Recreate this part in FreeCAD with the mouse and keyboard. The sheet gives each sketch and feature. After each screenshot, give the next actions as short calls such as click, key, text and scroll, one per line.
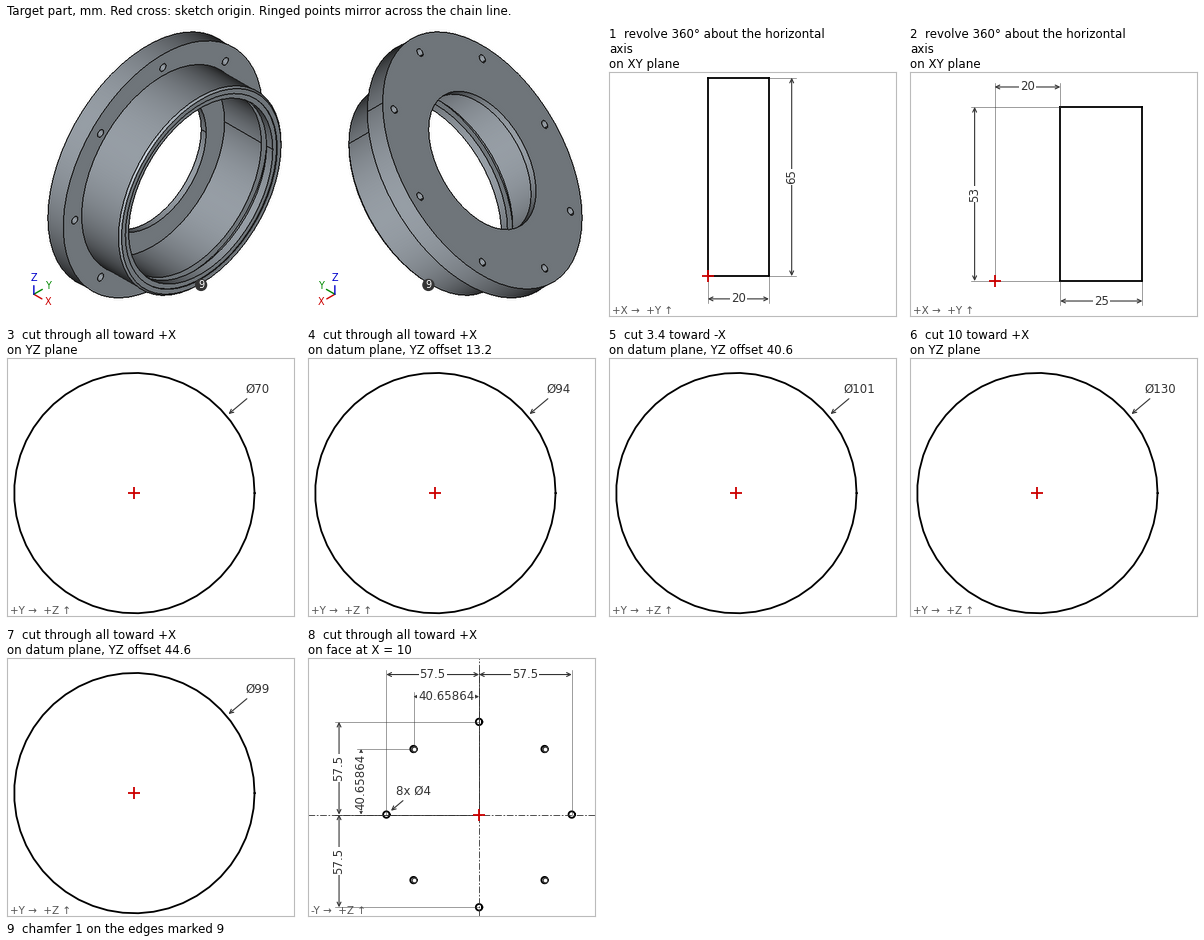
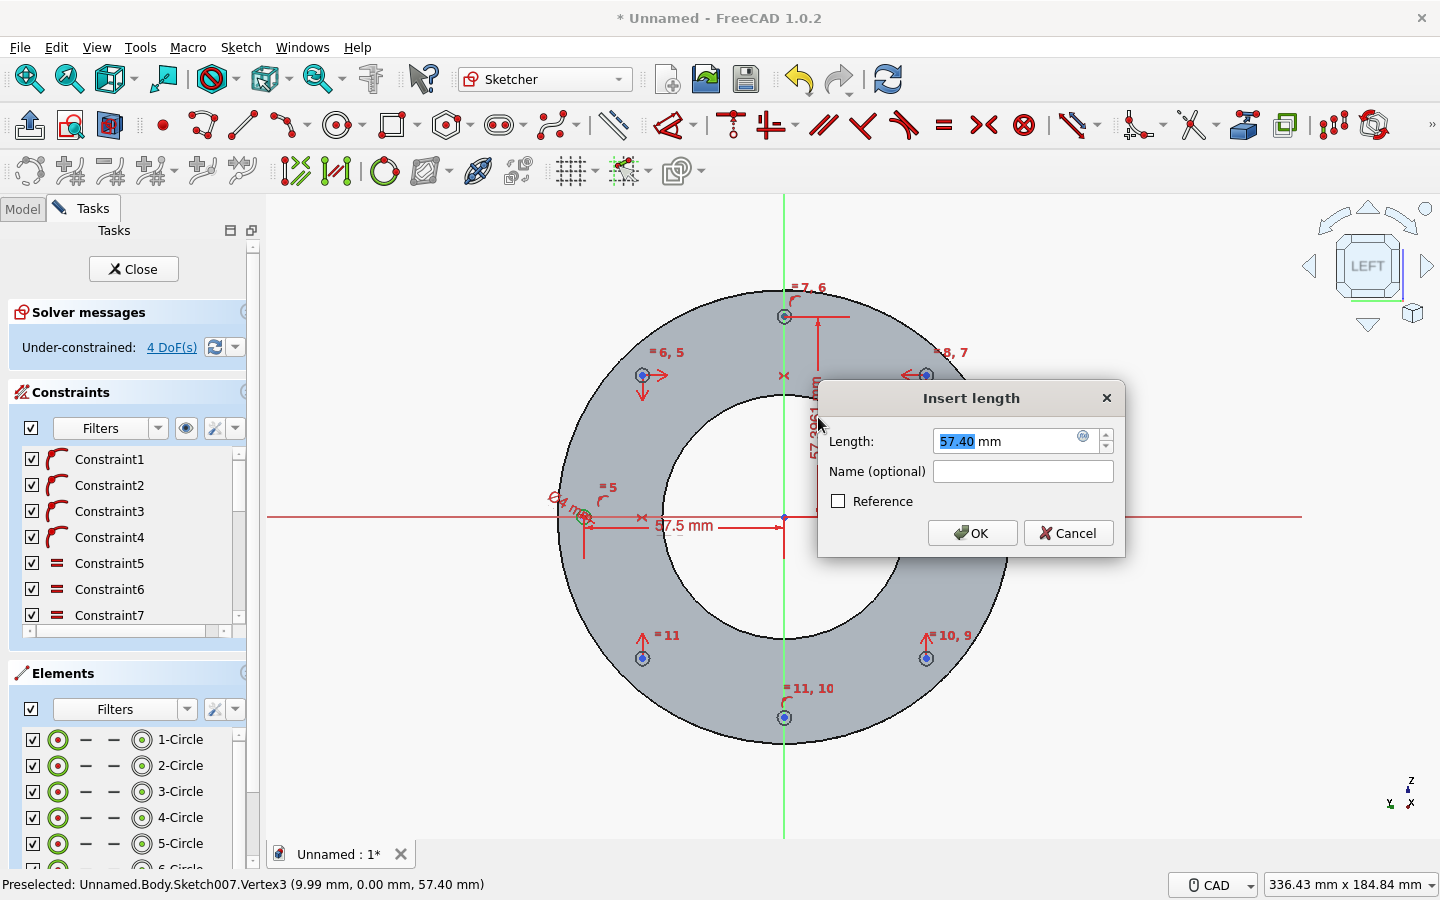
text(57.5)
key(Return)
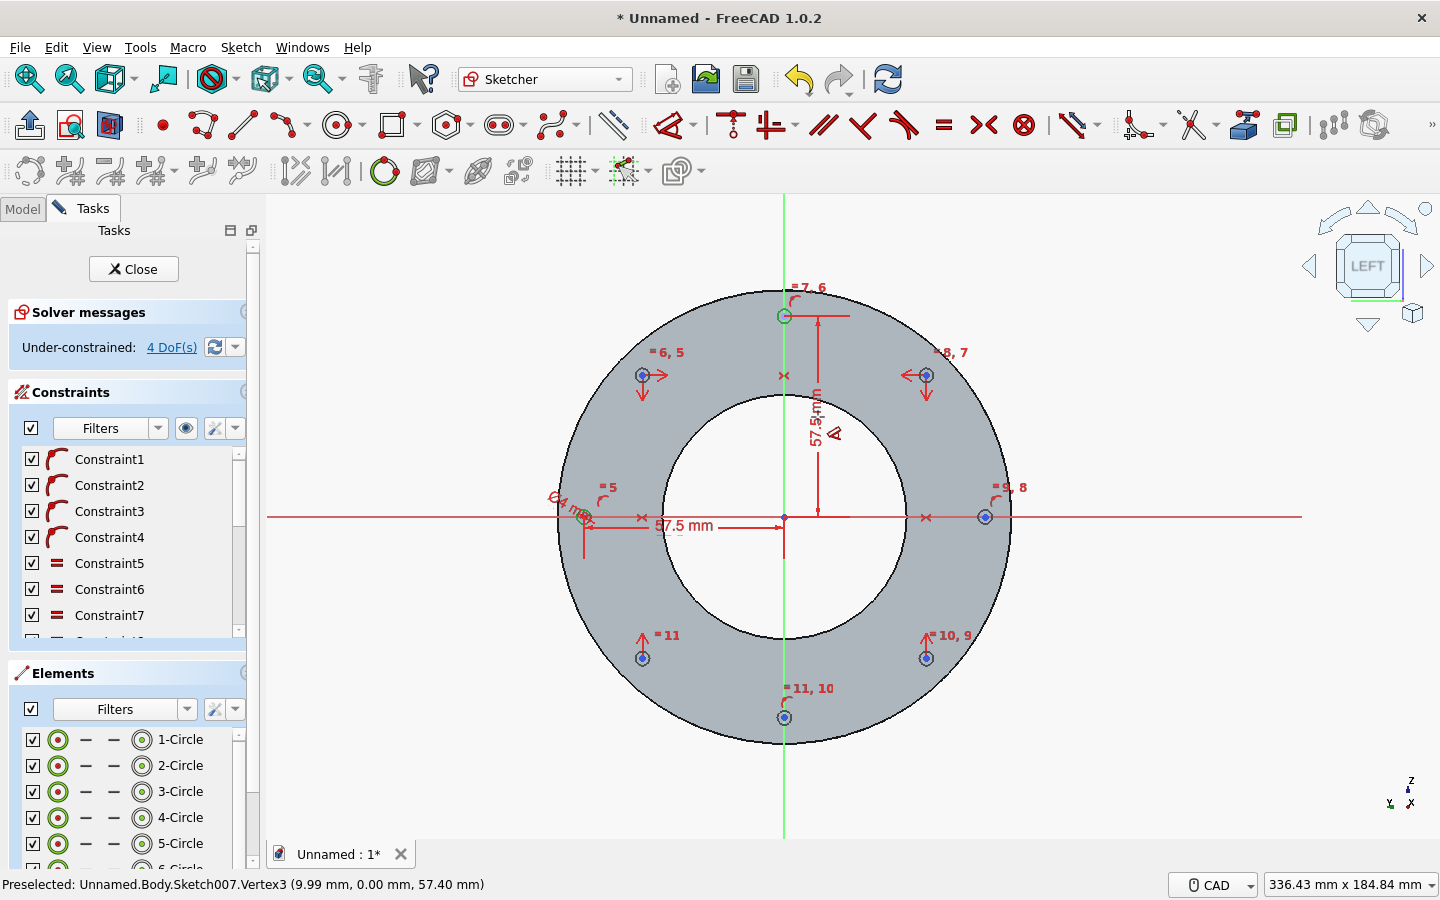
click(985, 517)
click(885, 551)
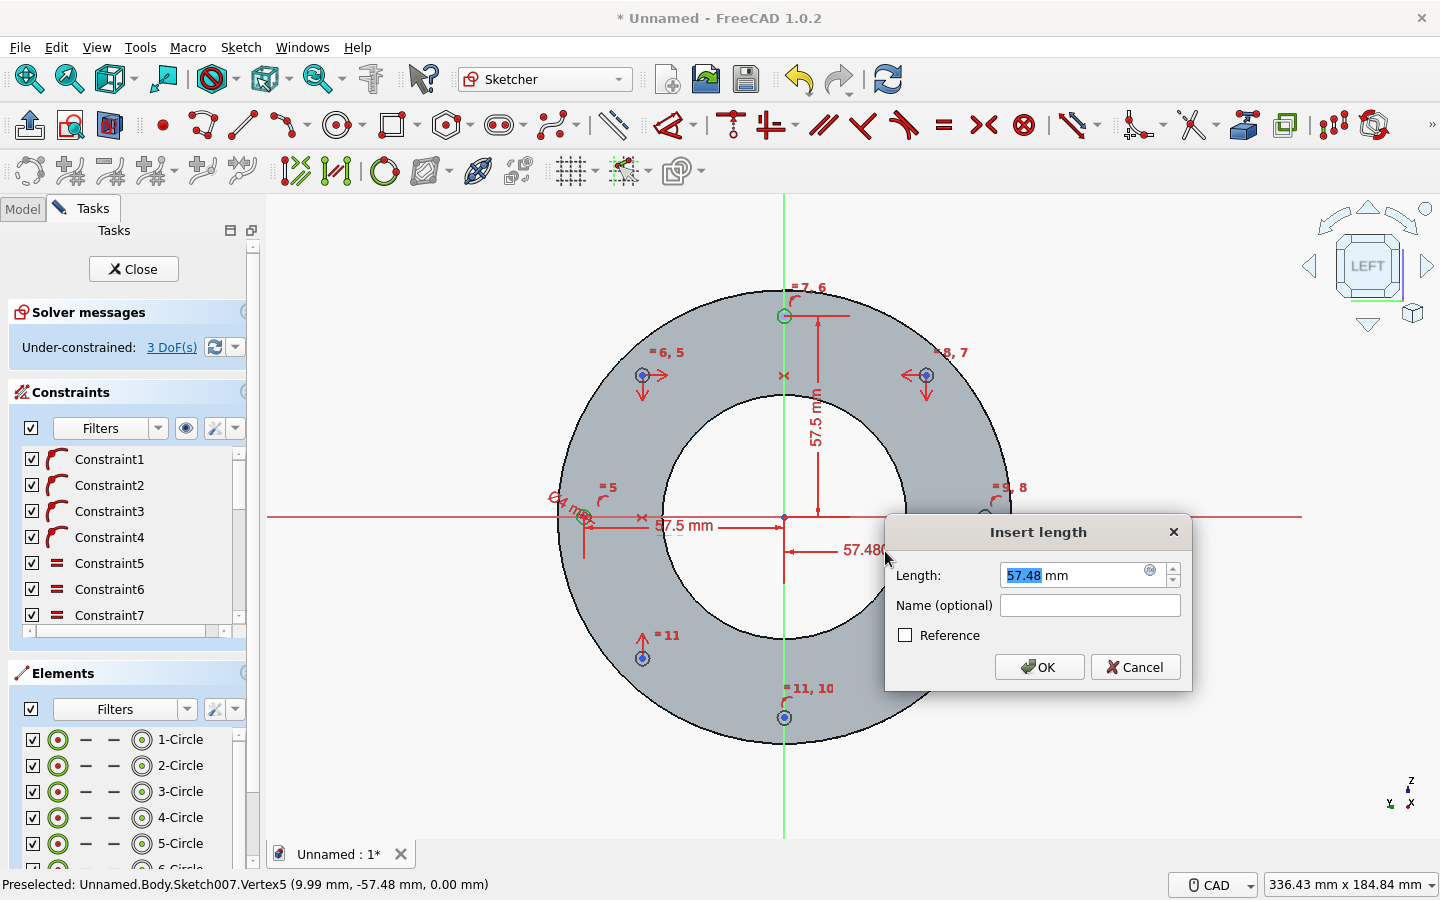
text(57.5)
key(Return)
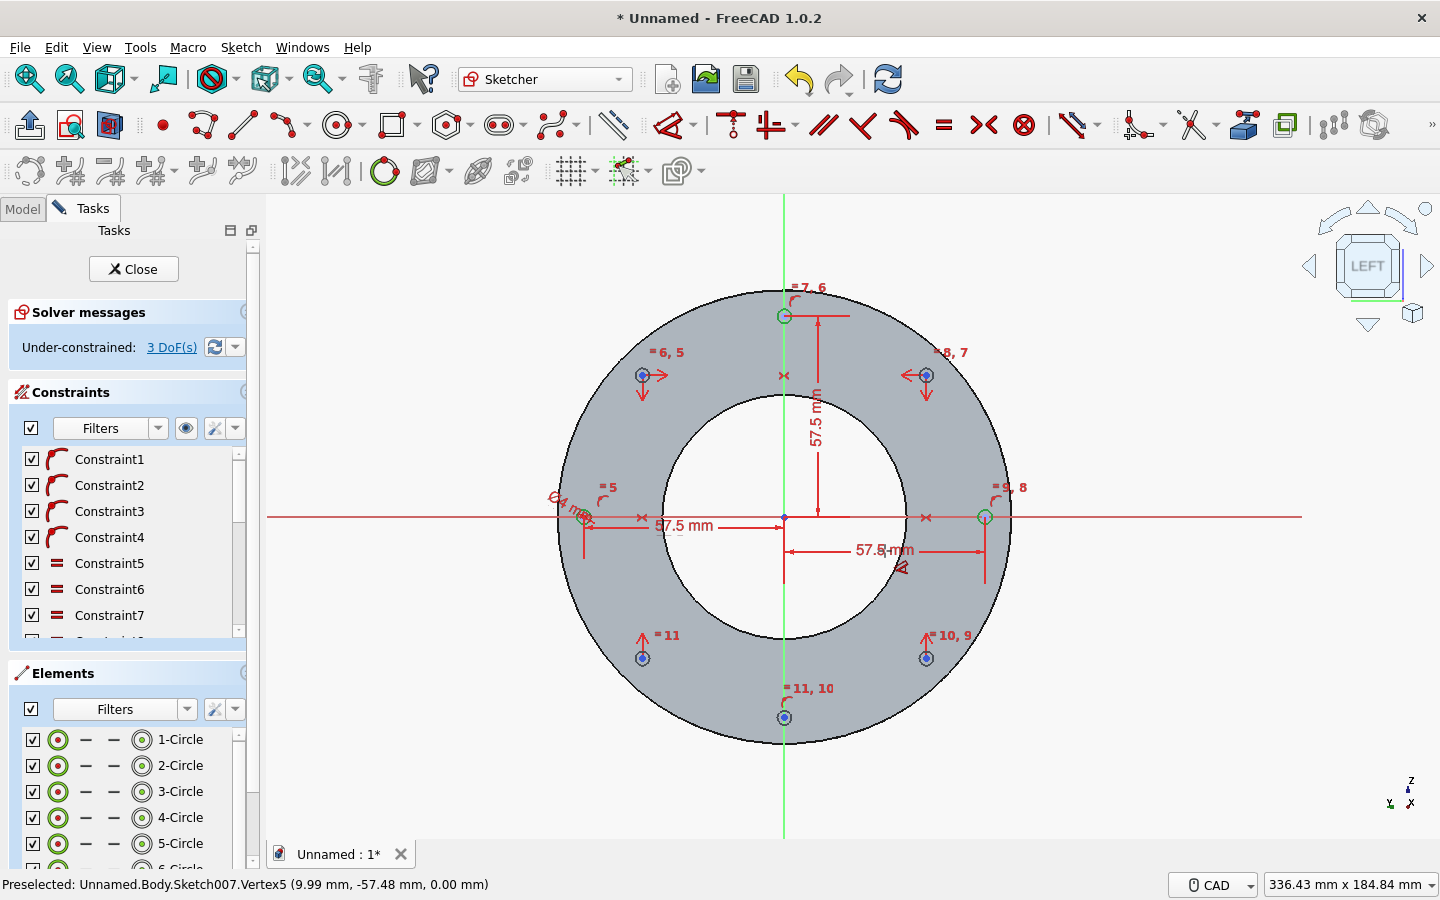
click(784, 718)
click(818, 617)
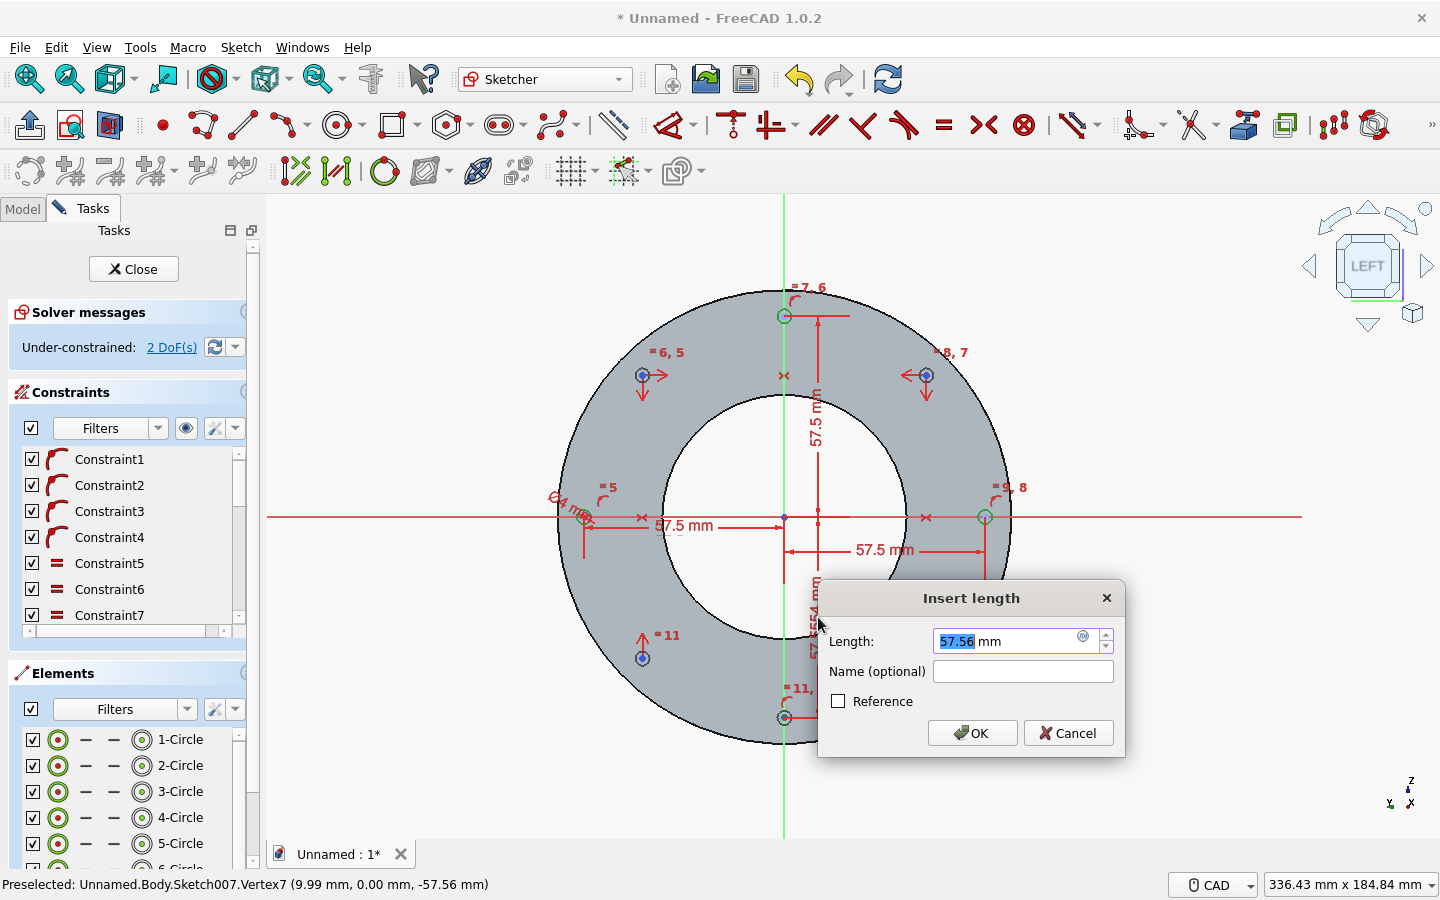
text(57.5)
key(Return)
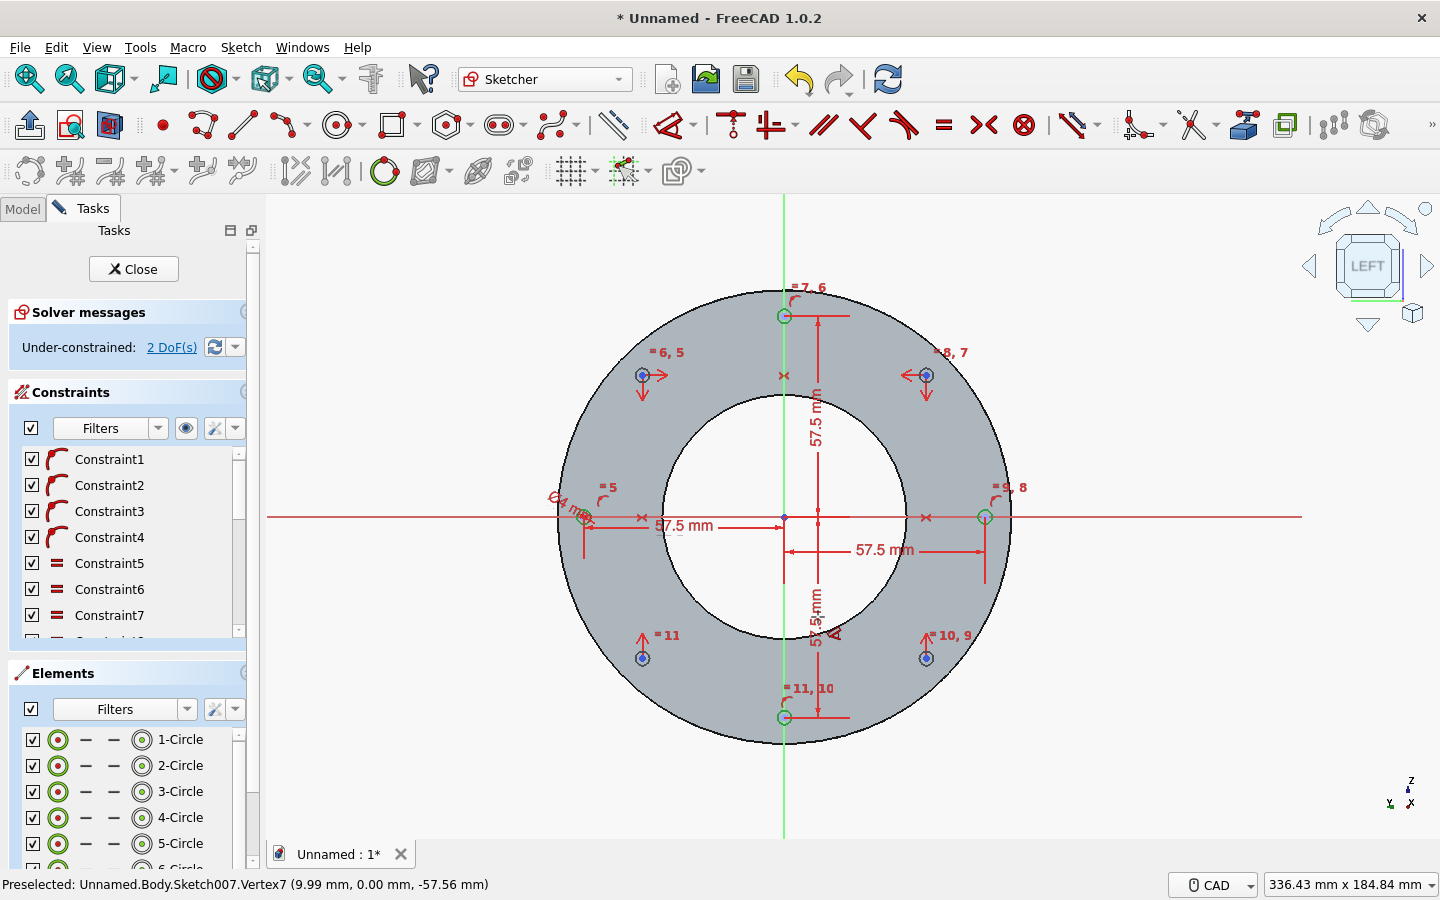
click(643, 375)
click(714, 341)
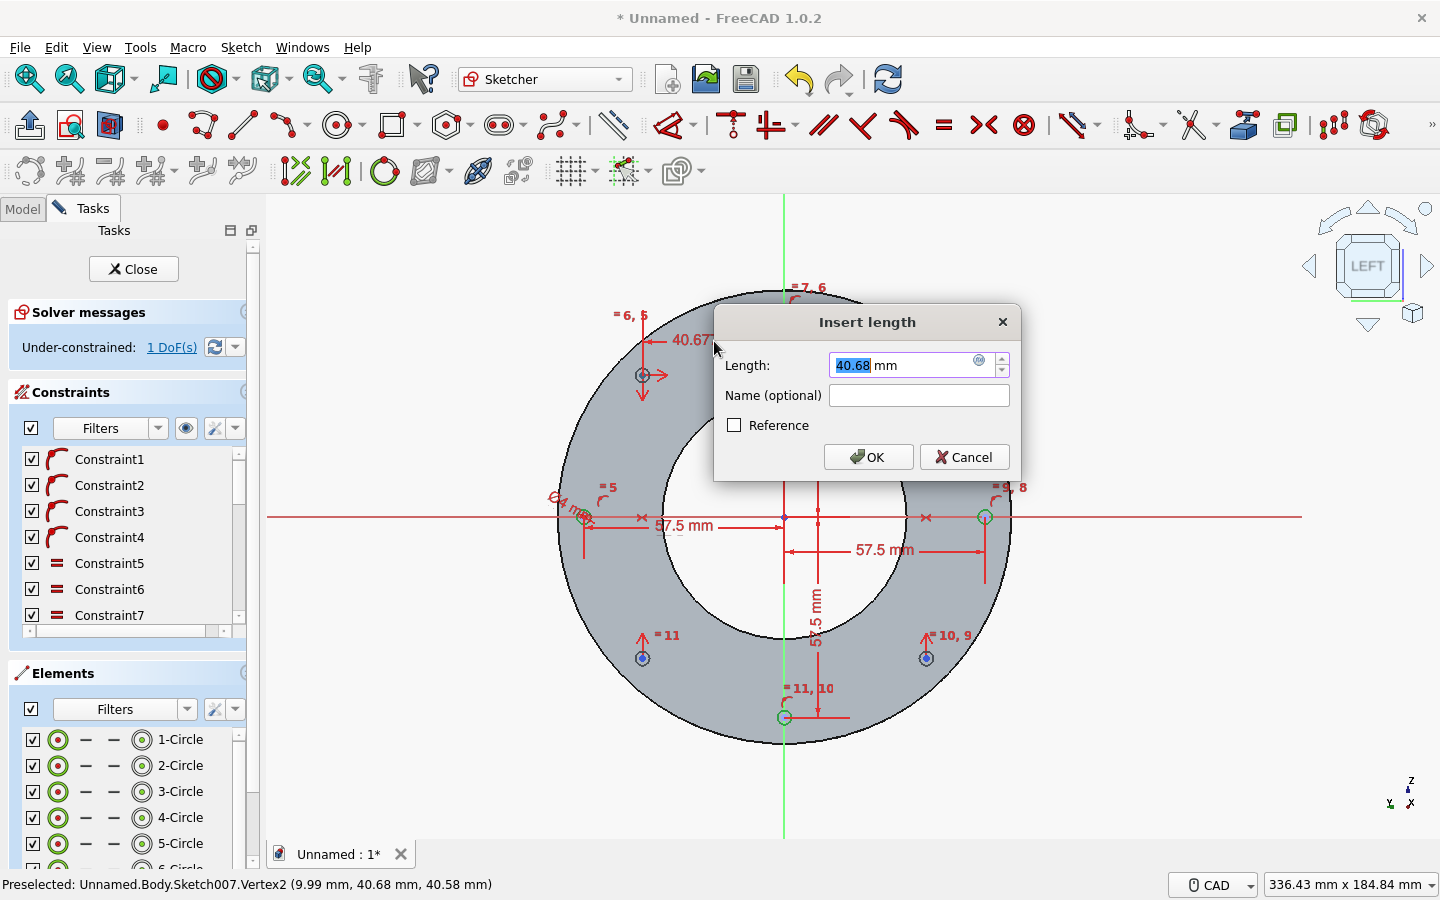
text(40.65864)
key(Return)